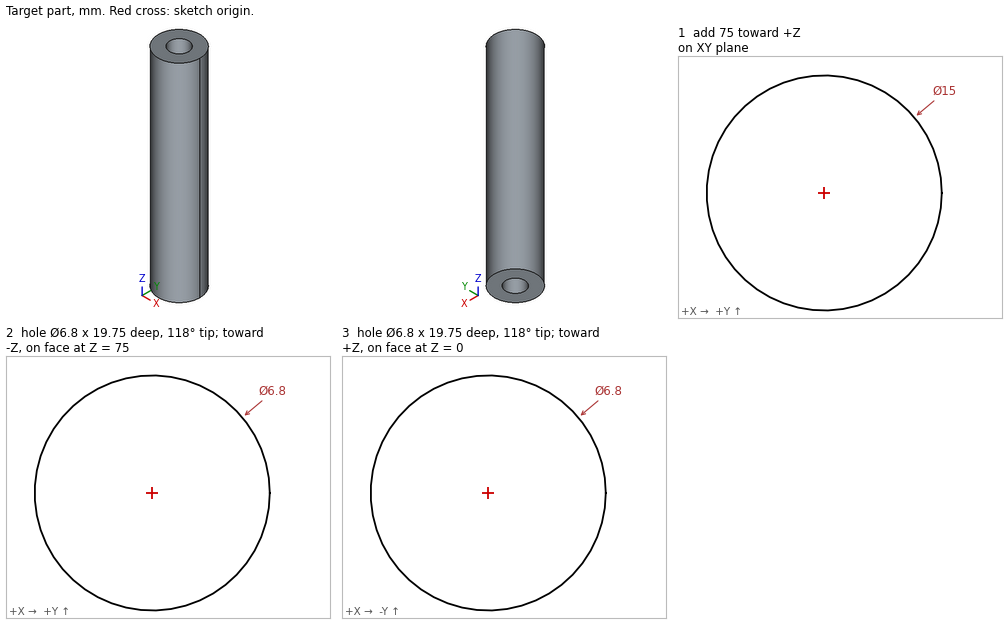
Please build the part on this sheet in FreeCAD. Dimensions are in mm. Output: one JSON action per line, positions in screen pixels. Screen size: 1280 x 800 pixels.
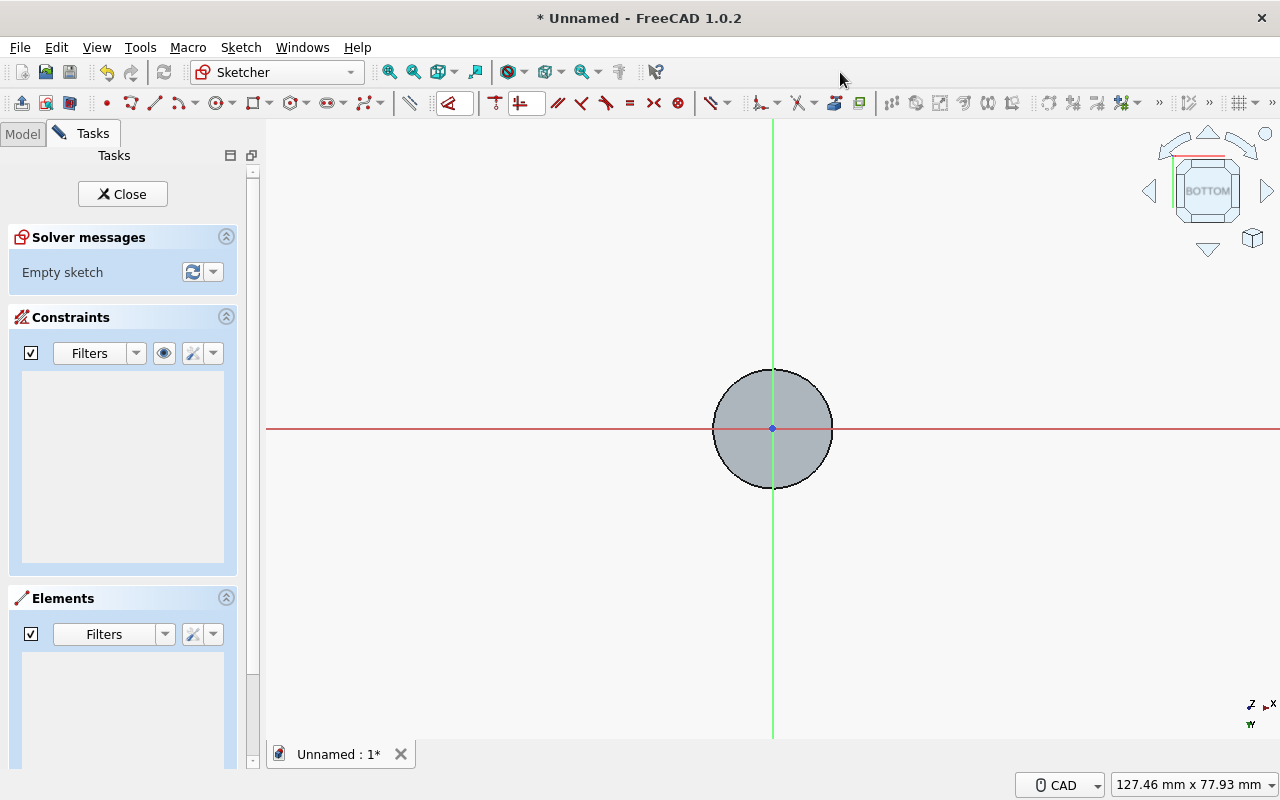
{"action": "scroll", "coordinate": [784, 429], "scroll_direction": "up", "scroll_amount": 10}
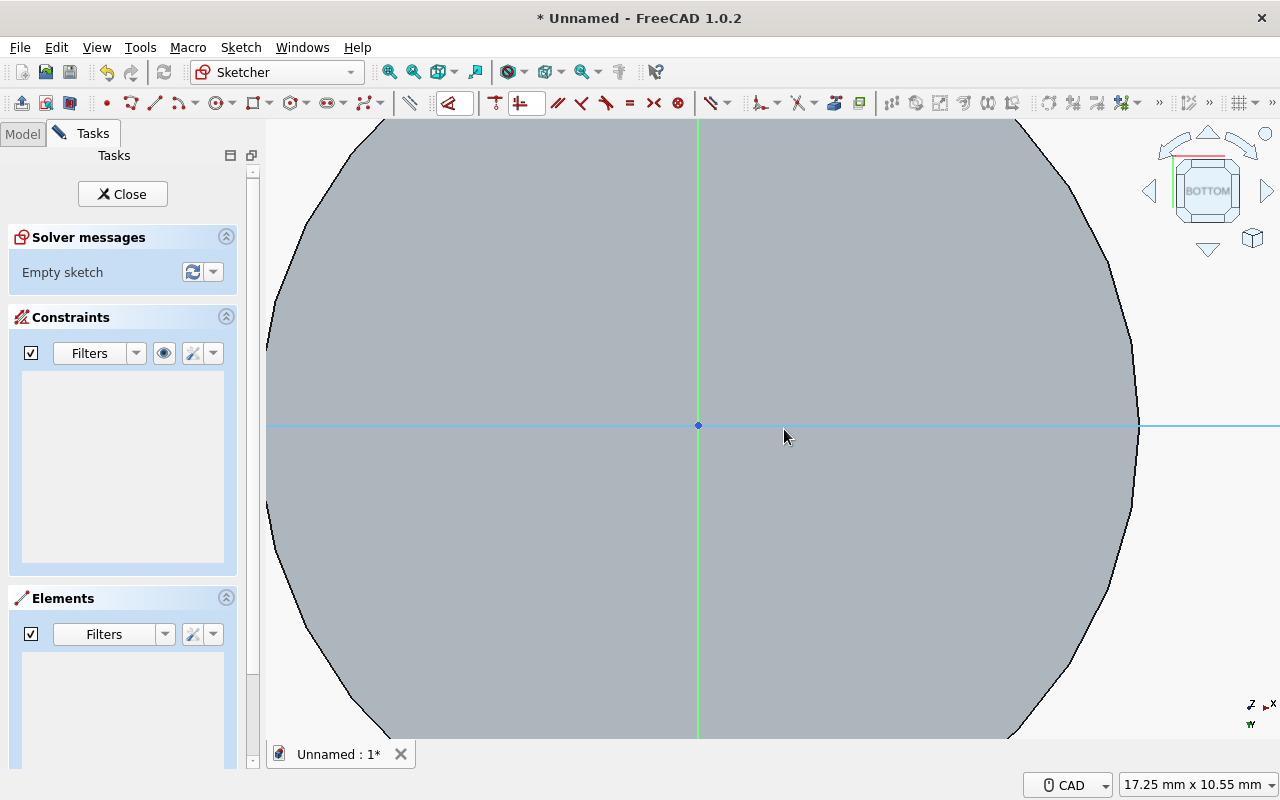
{"action": "left_click", "coordinate": [216, 104]}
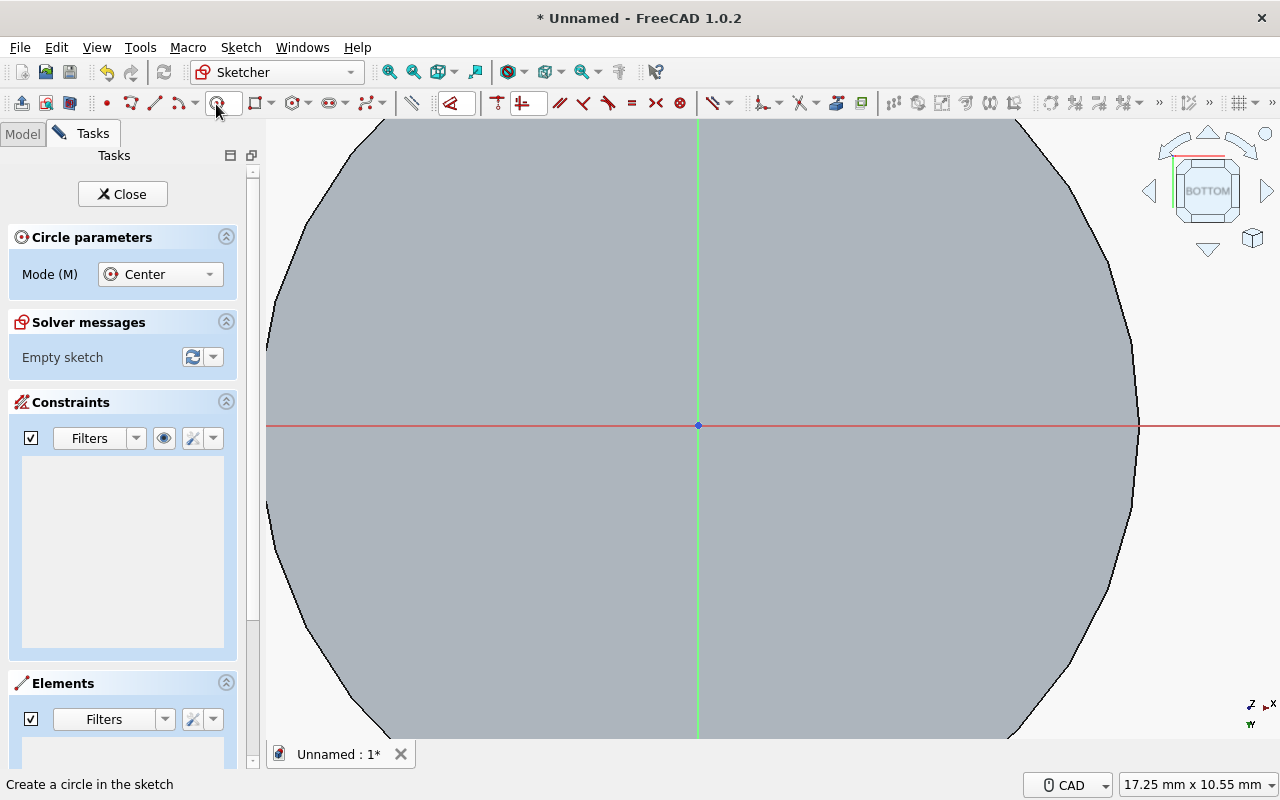
{"action": "left_click", "coordinate": [698, 426]}
{"action": "mouse_move", "coordinate": [840, 284]}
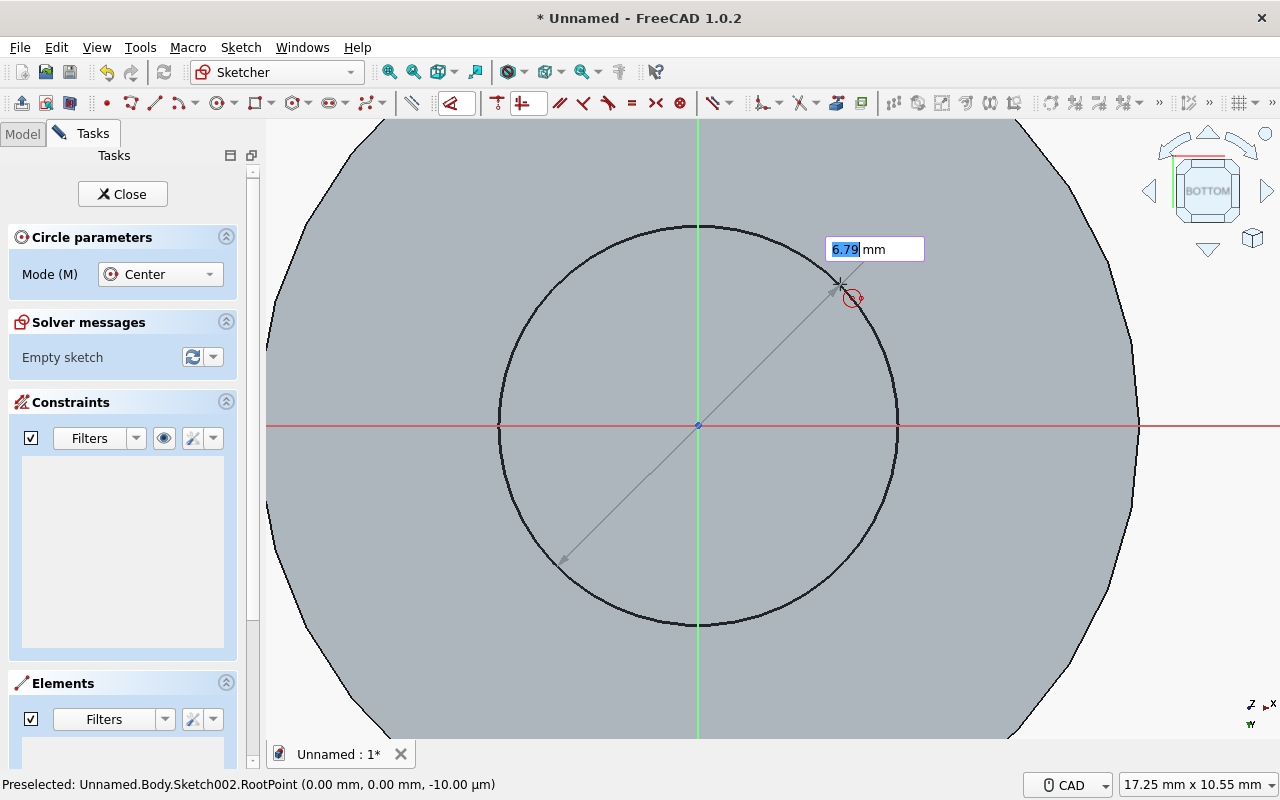
{"action": "type", "text": "6.8"}
{"action": "key", "text": "Return"}
{"action": "key", "text": "Escape"}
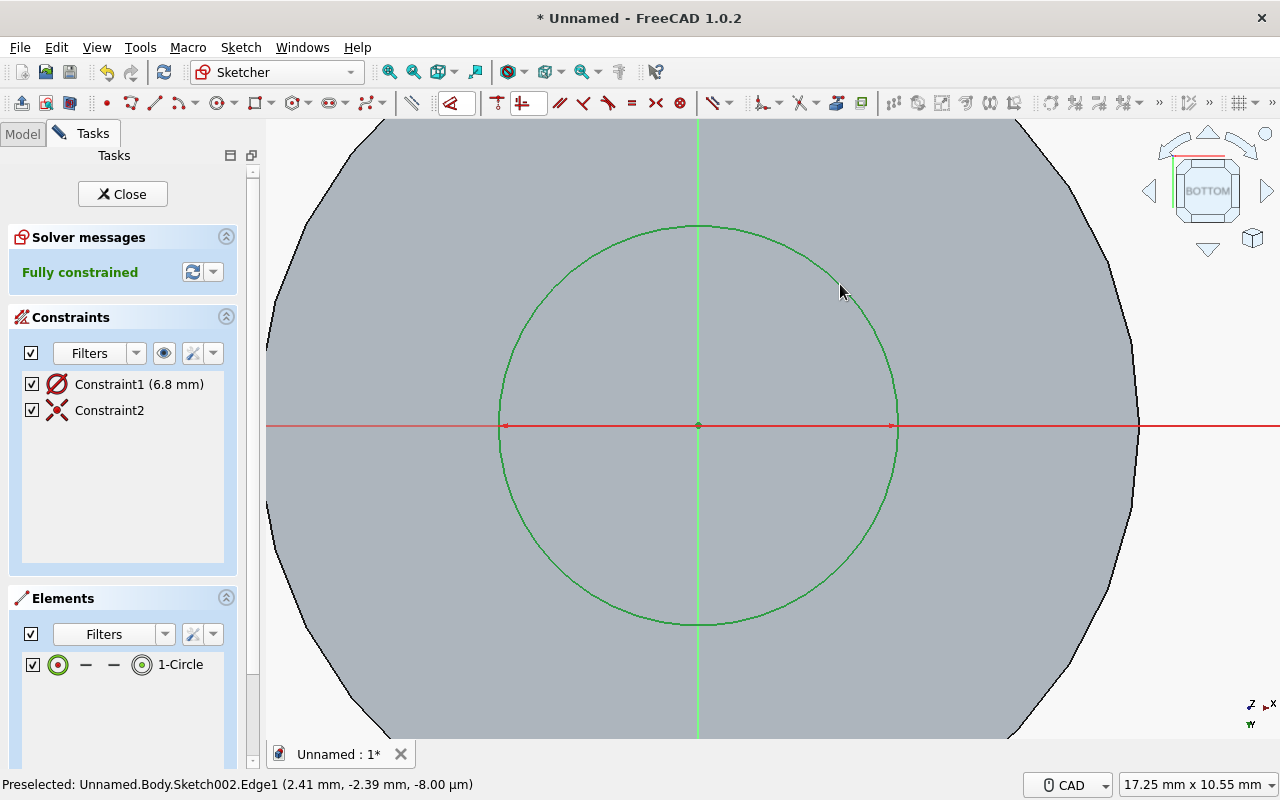
{"action": "left_click", "coordinate": [123, 194]}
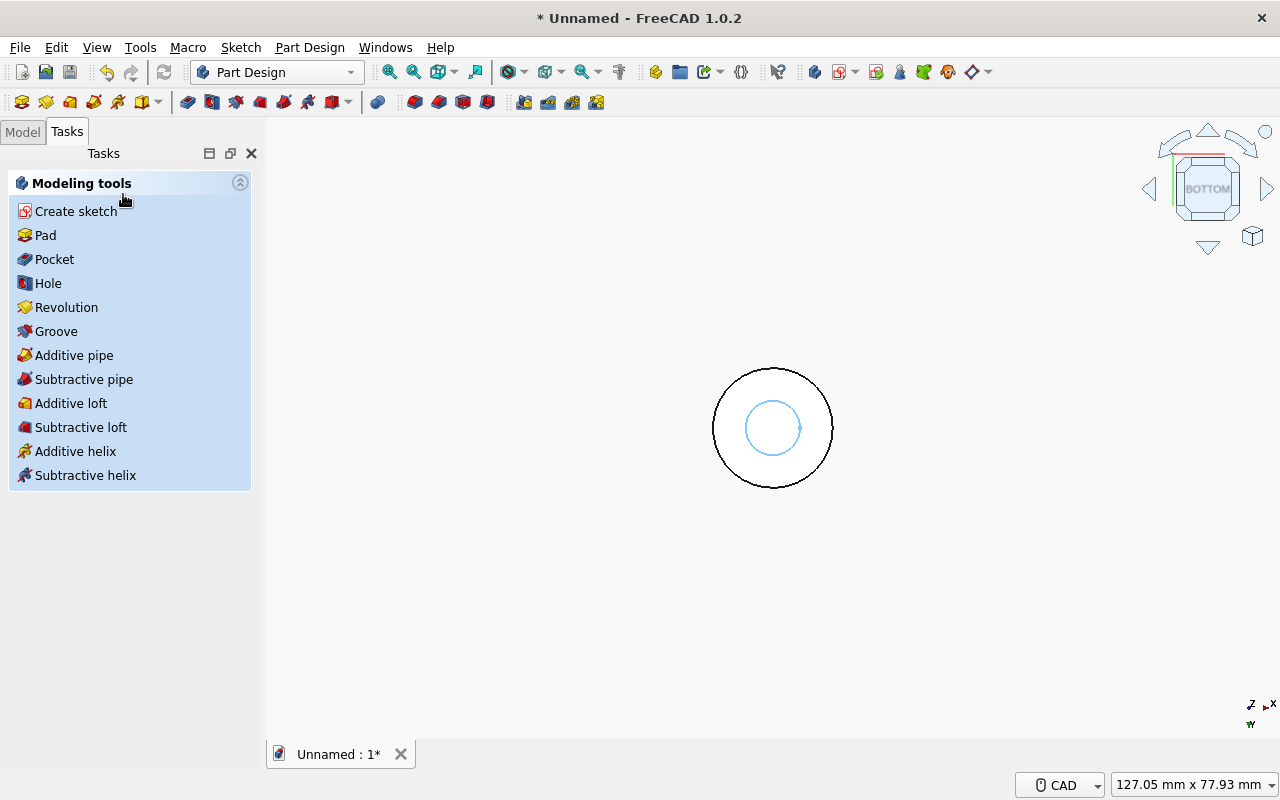
{"action": "left_click", "coordinate": [212, 102]}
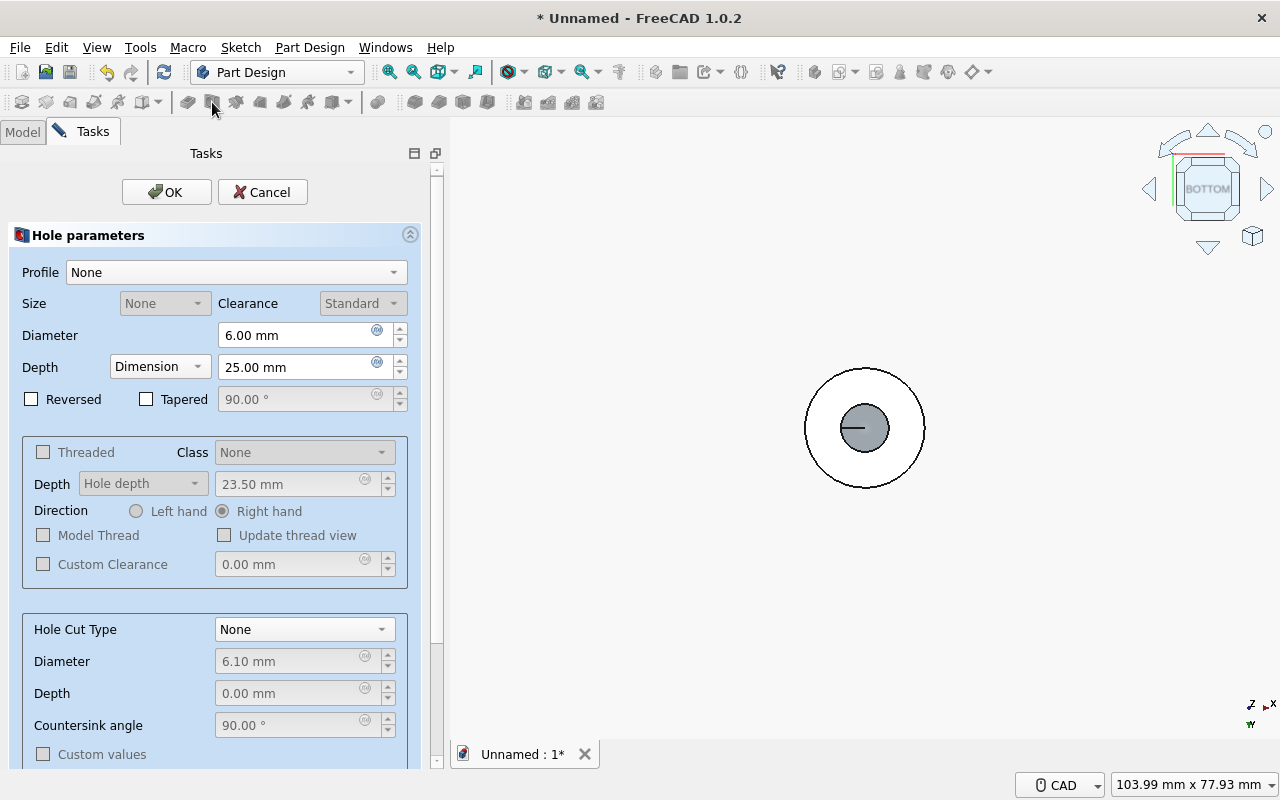
{"action": "triple_click", "coordinate": [305, 335]}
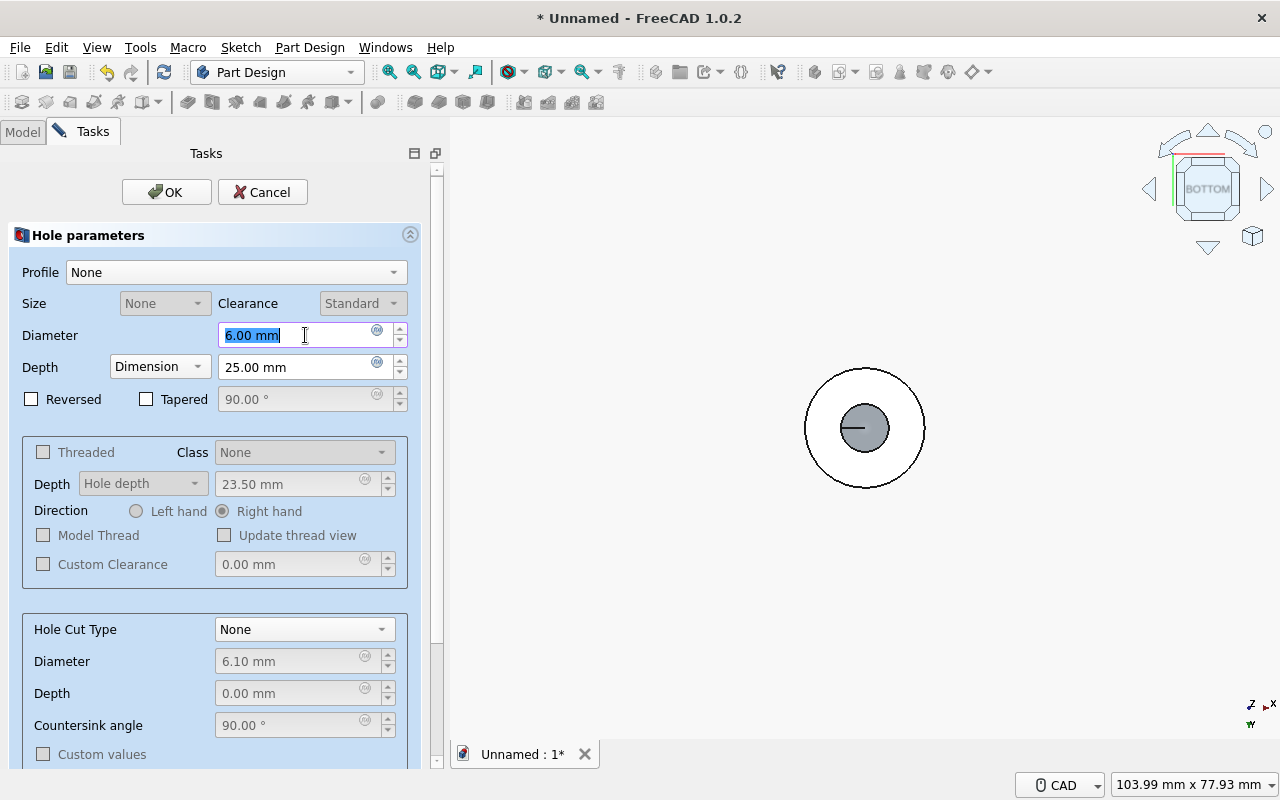
{"action": "type", "text": "6.8"}
{"action": "key", "text": "Tab"}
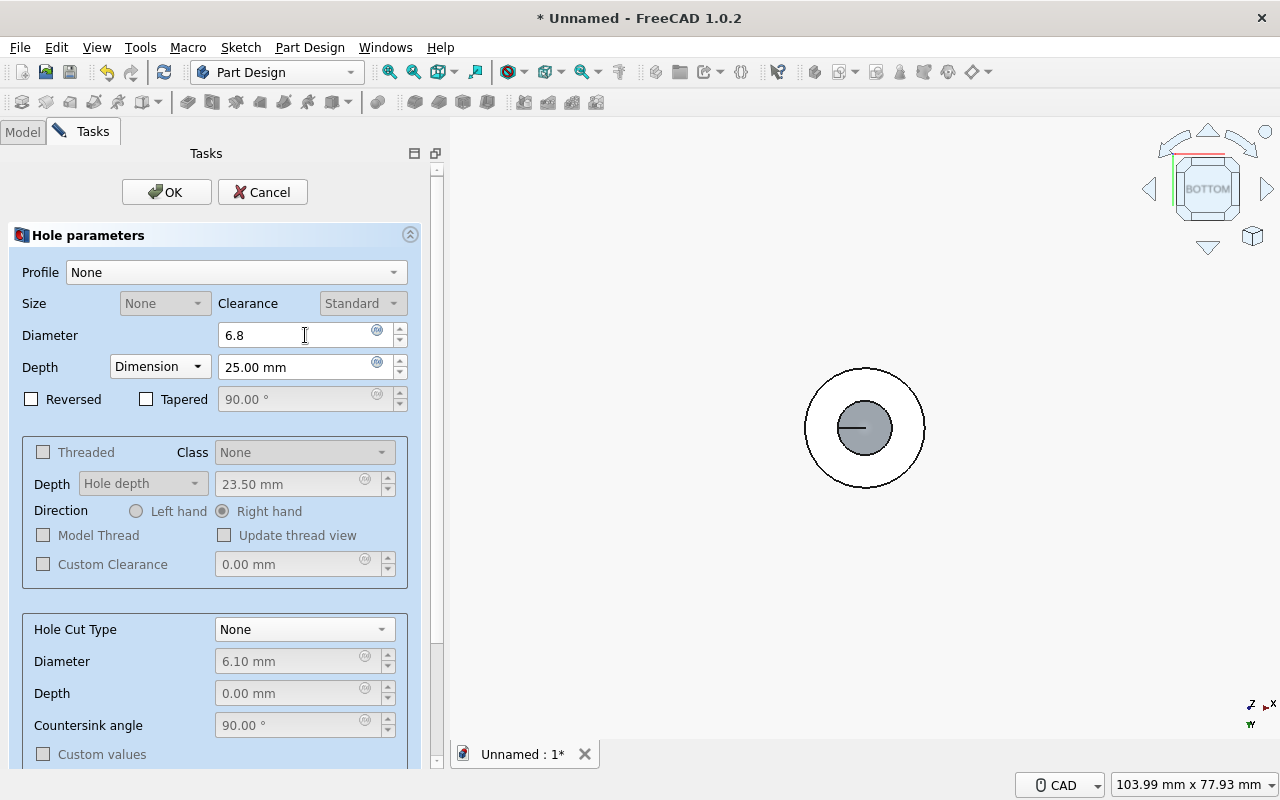
{"action": "triple_click", "coordinate": [305, 367]}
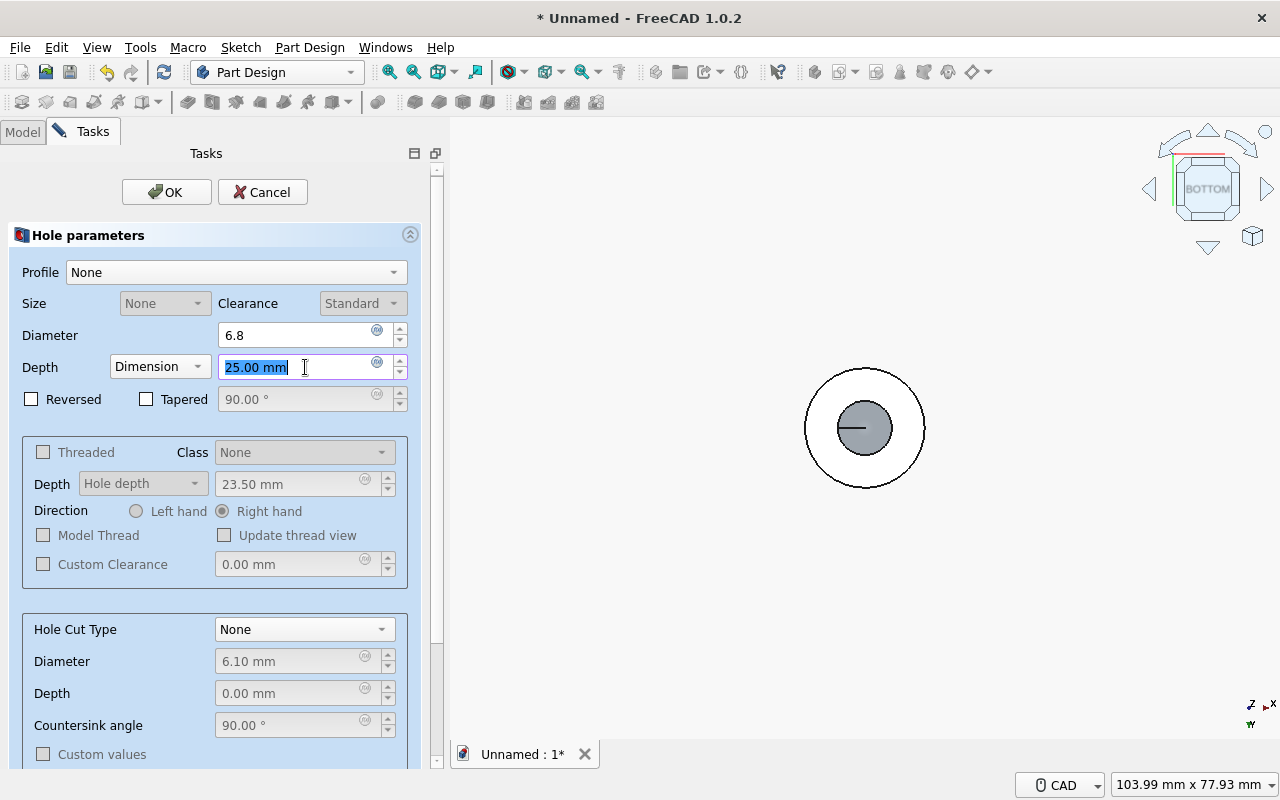
{"action": "type", "text": "19.75"}
{"action": "key", "text": "Tab"}